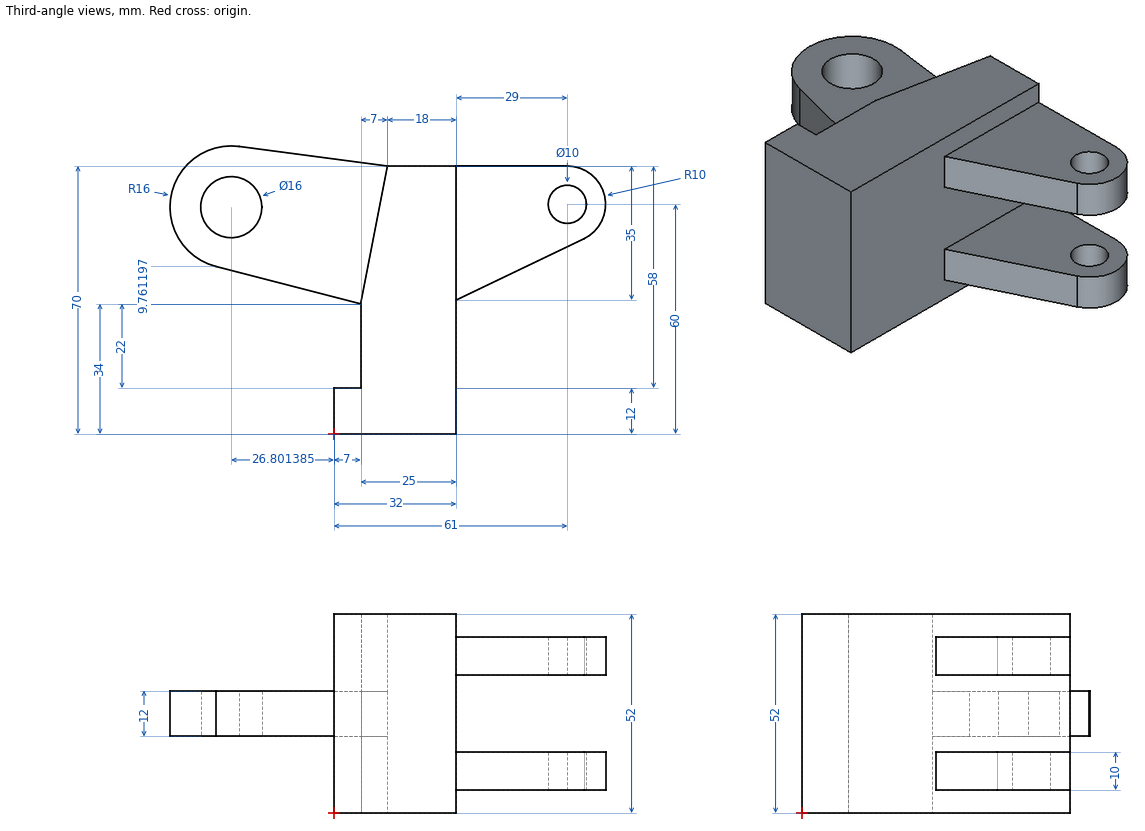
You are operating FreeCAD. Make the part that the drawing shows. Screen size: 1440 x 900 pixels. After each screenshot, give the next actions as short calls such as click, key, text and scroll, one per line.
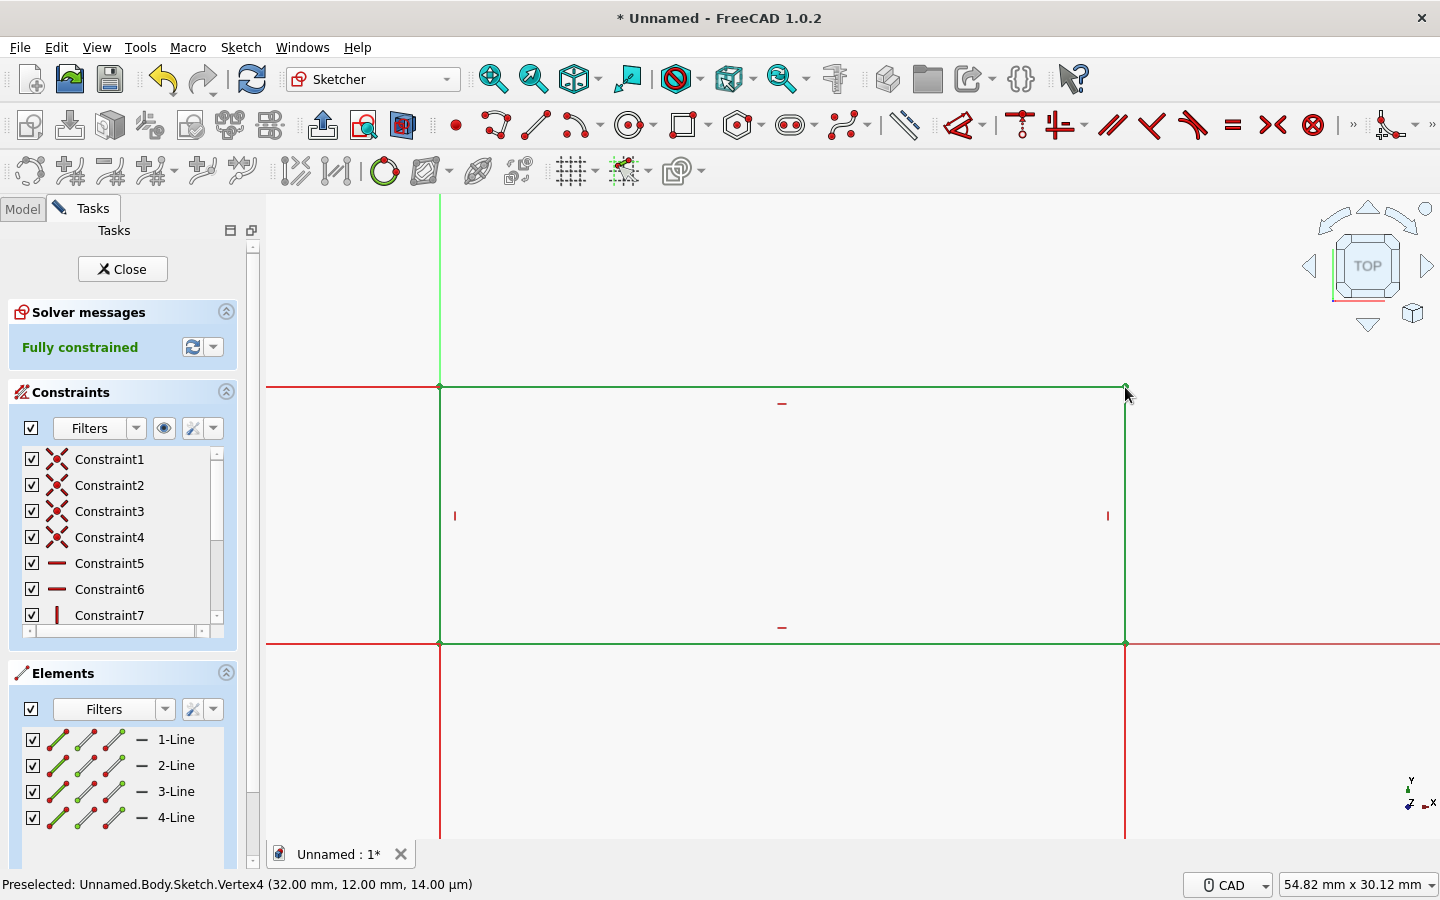
click(123, 269)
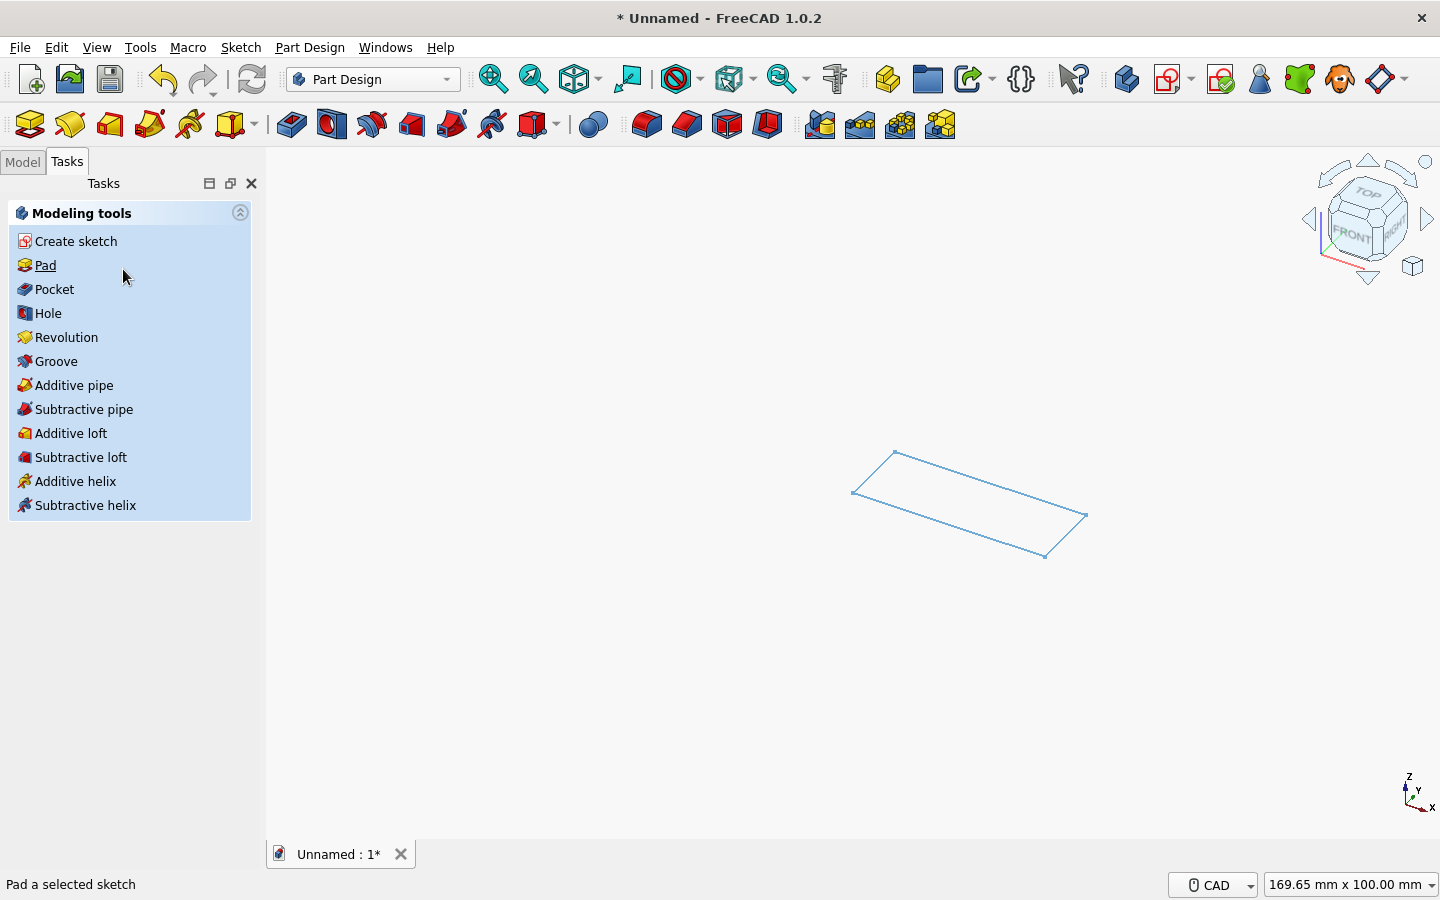
click(30, 124)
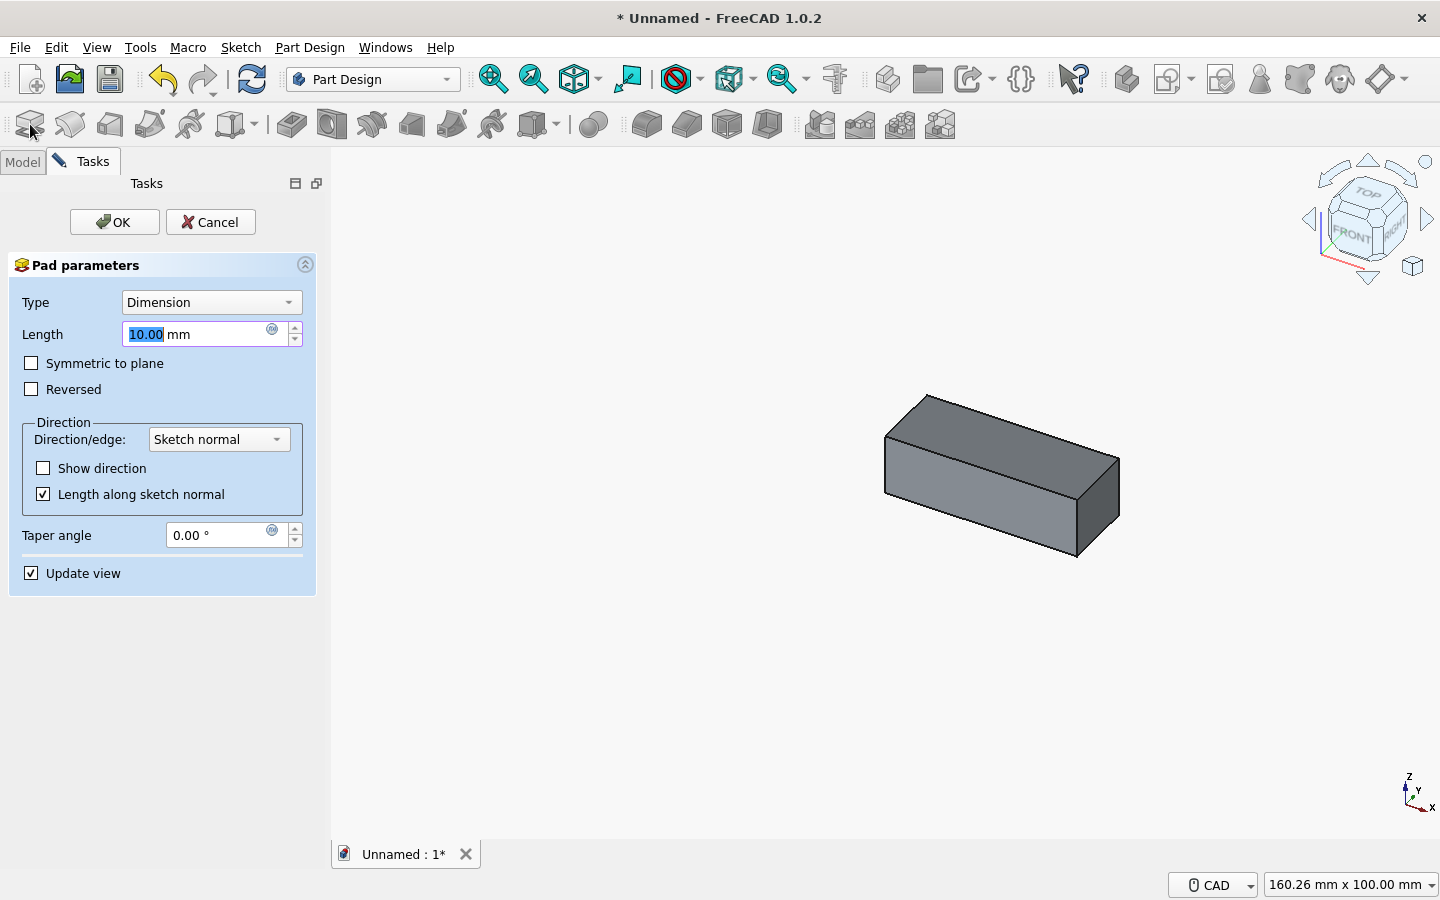
text(52)
key(Tab)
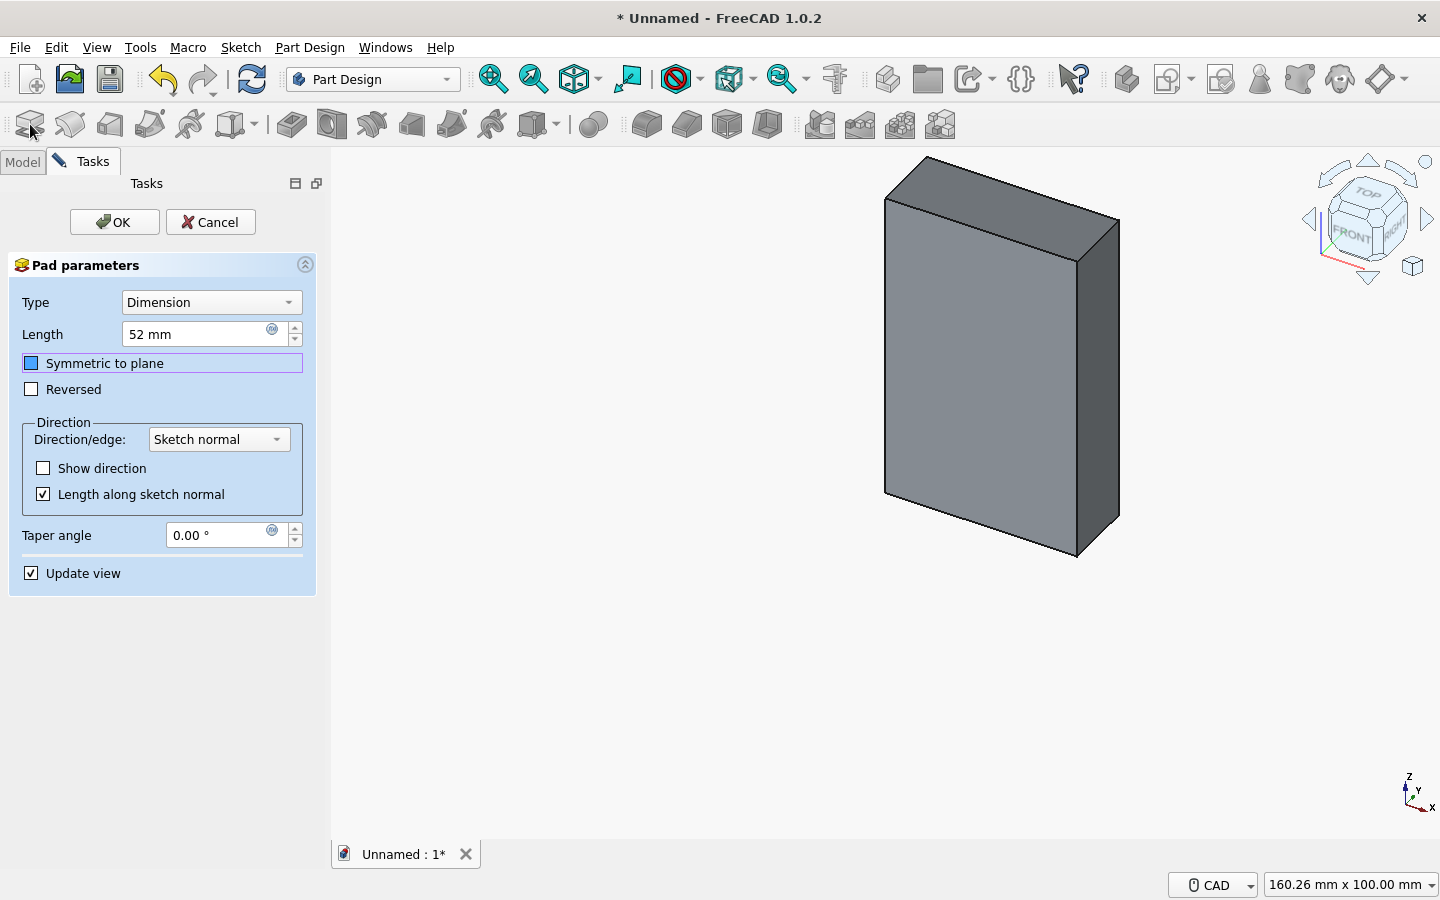
click(115, 222)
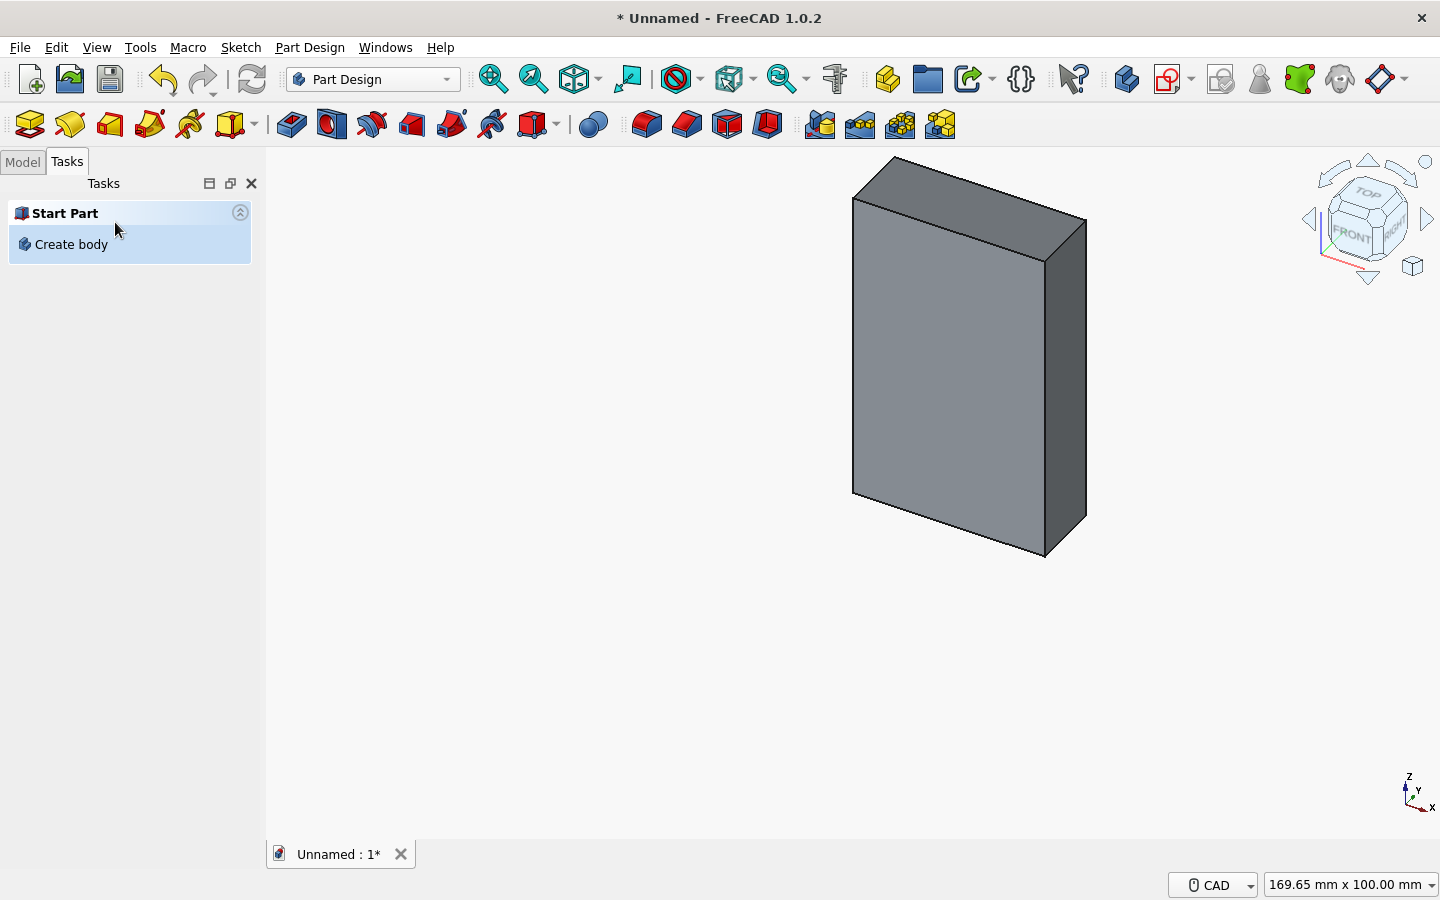
click(1024, 227)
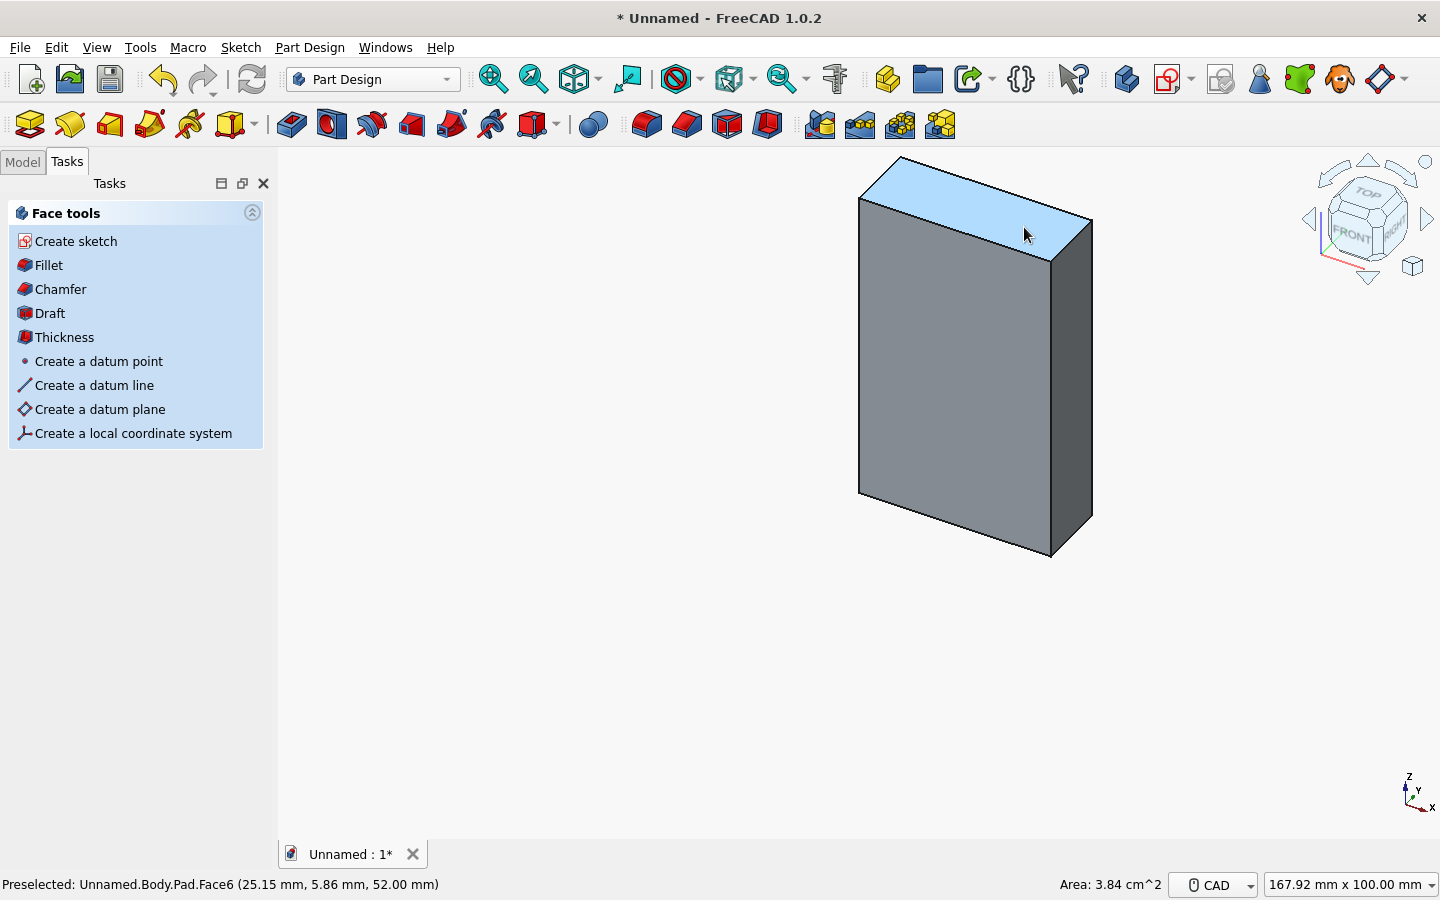
click(1168, 80)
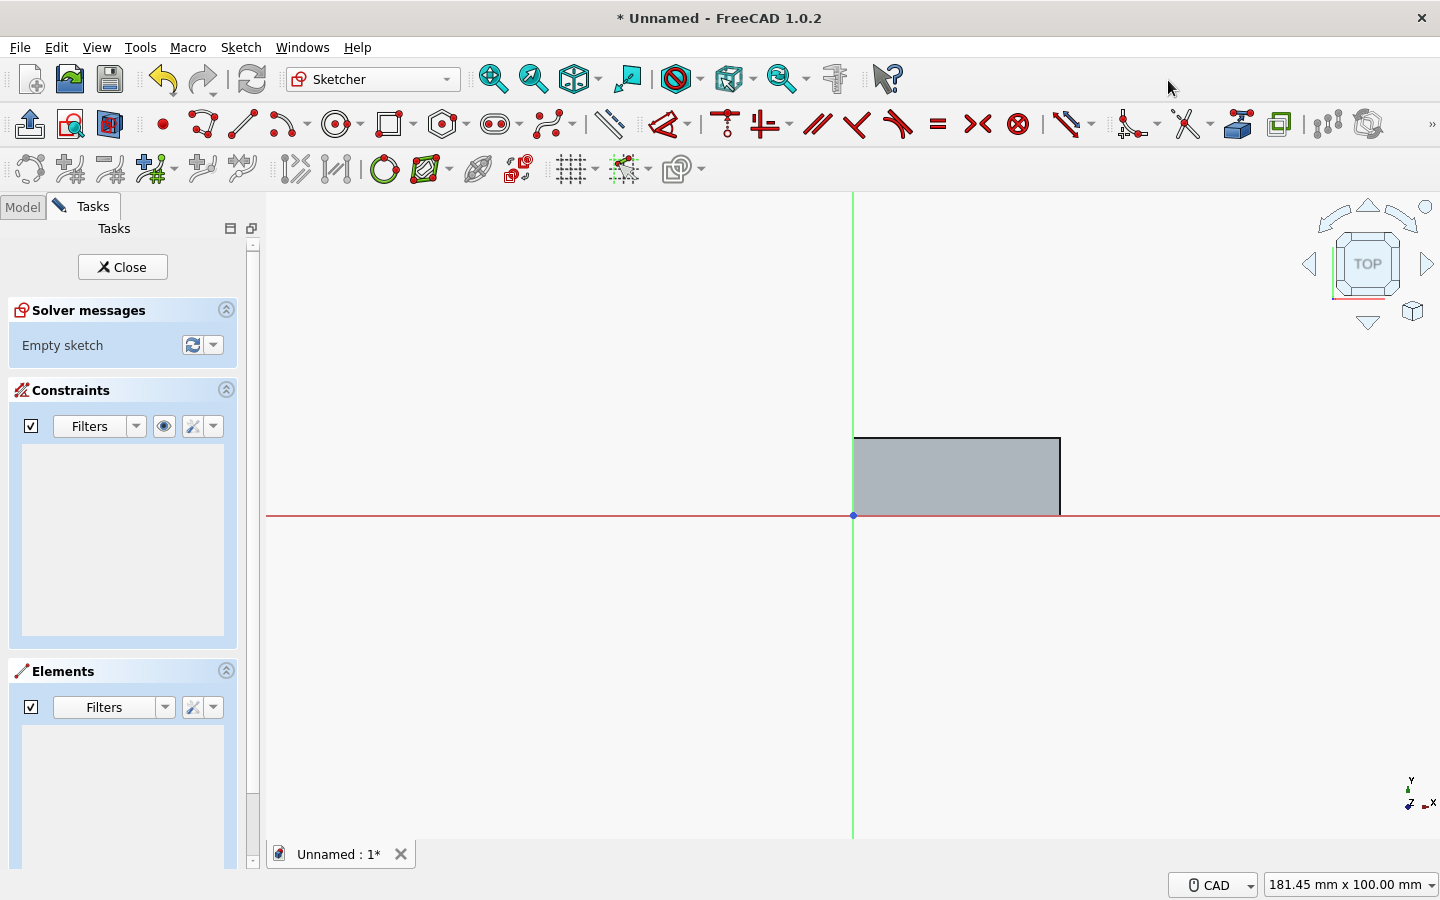
scroll(435, 811, down, 2)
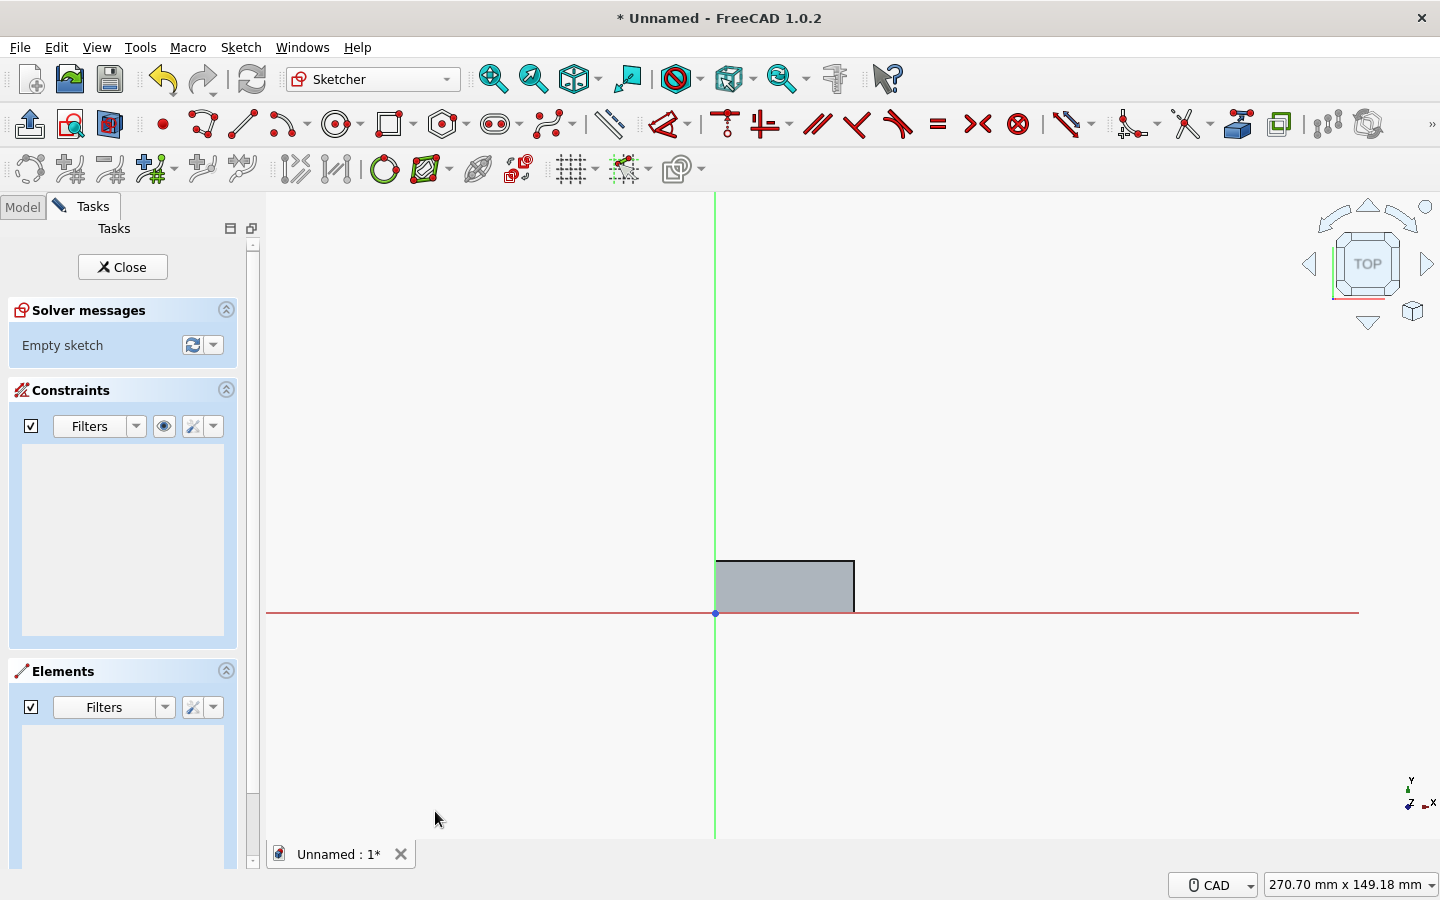
scroll(785, 352, up, 2)